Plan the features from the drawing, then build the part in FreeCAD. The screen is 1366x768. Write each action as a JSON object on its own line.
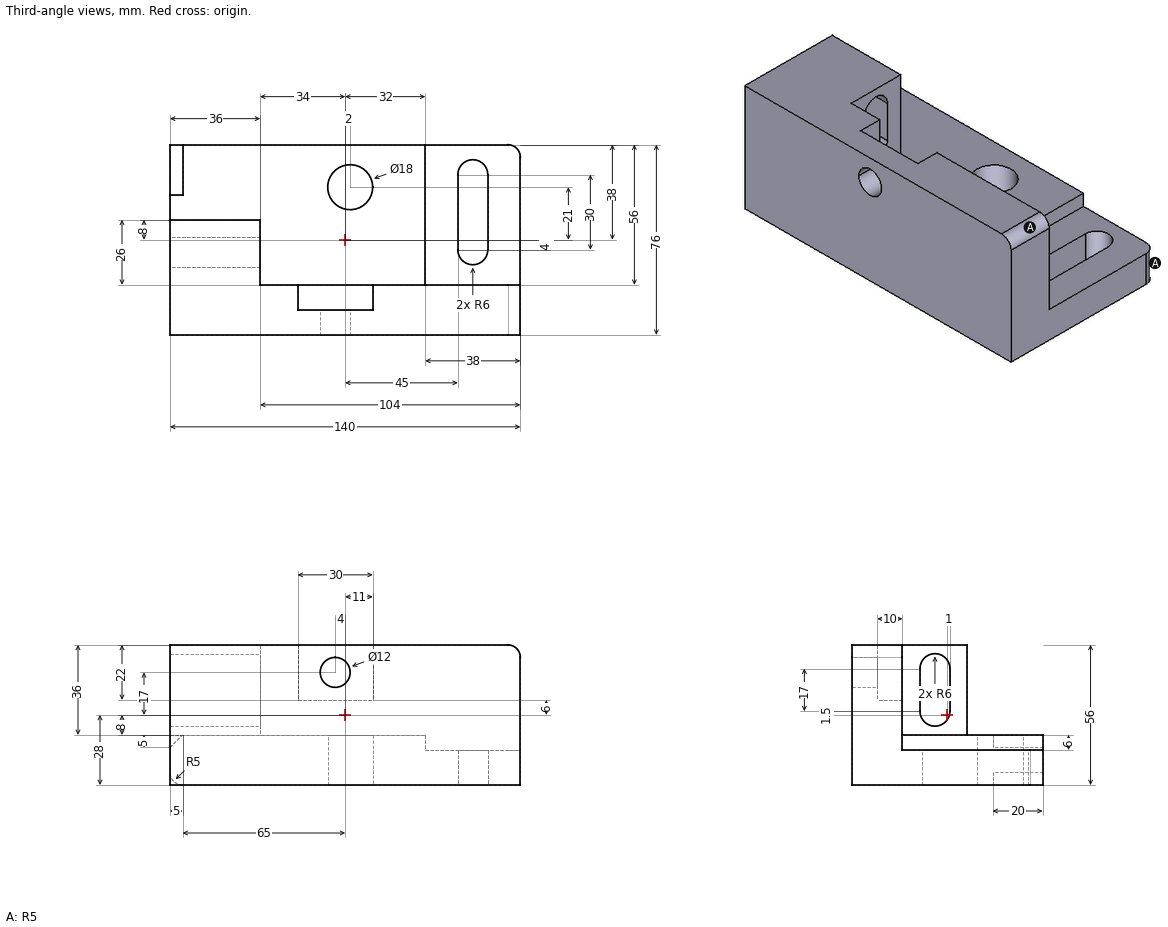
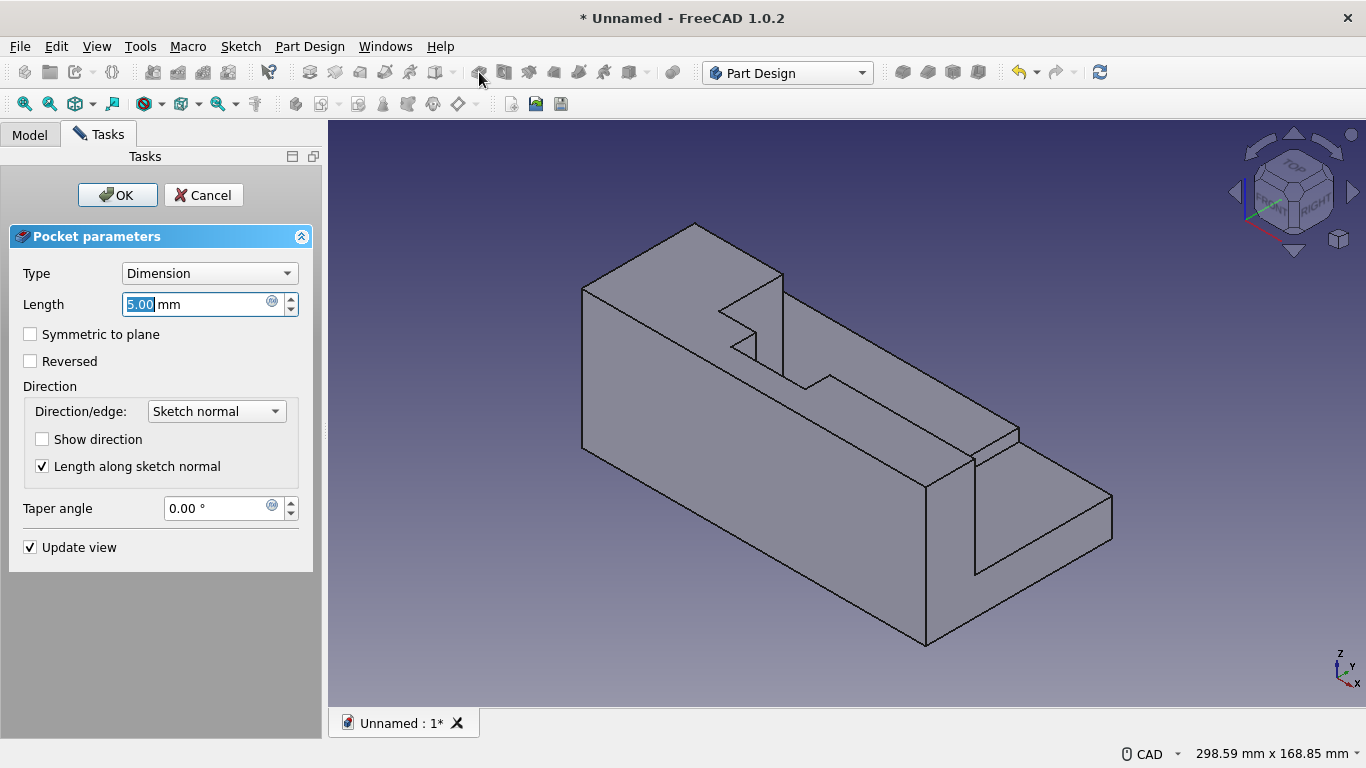
{"action": "type", "text": "6"}
{"action": "key", "text": "Tab"}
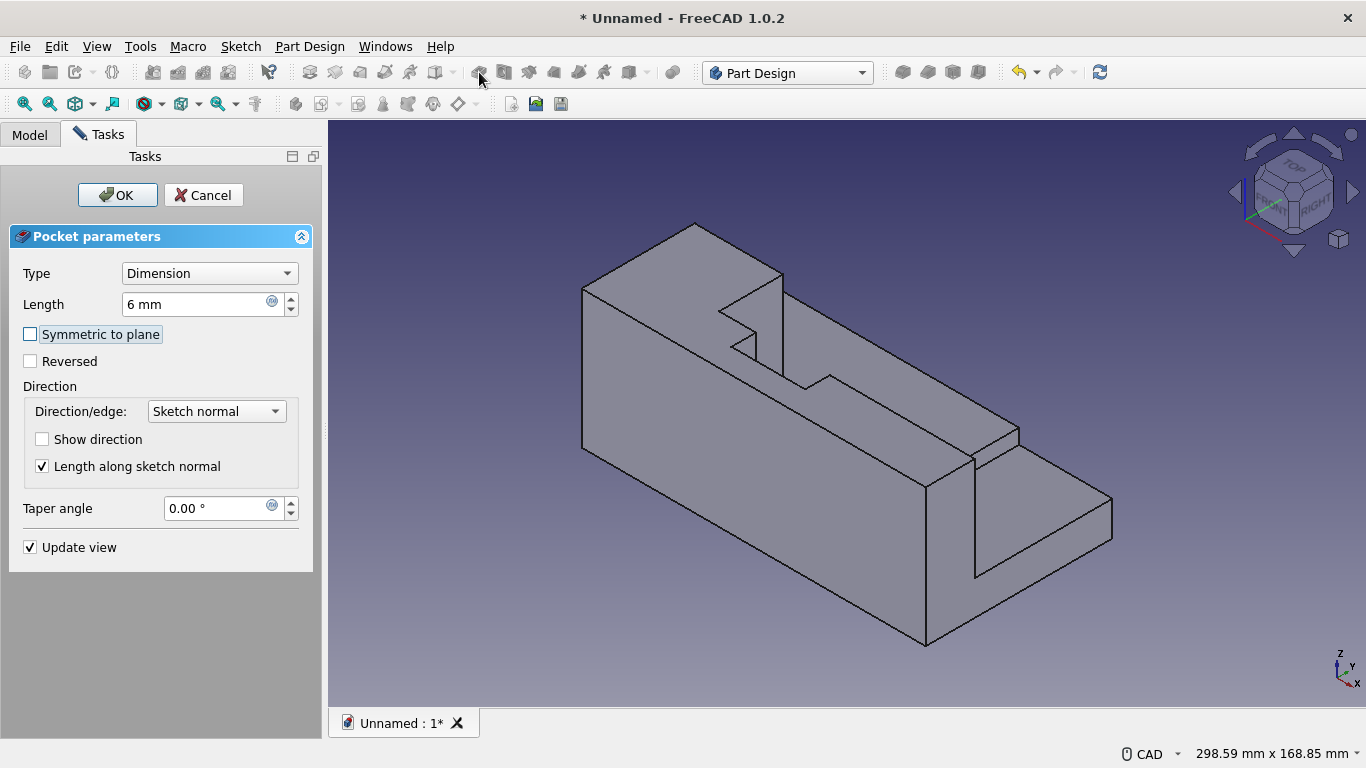
{"action": "left_click", "coordinate": [118, 195]}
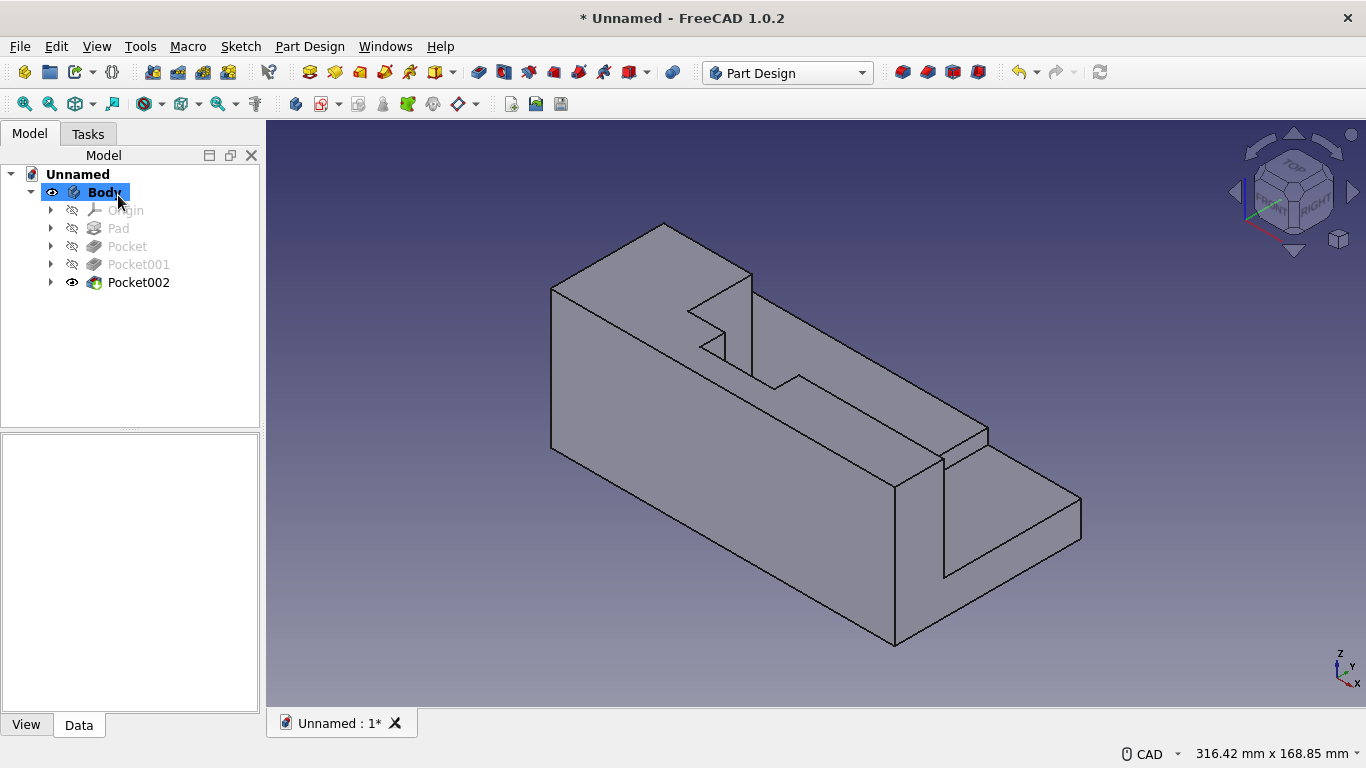
{"action": "key", "text": "2"}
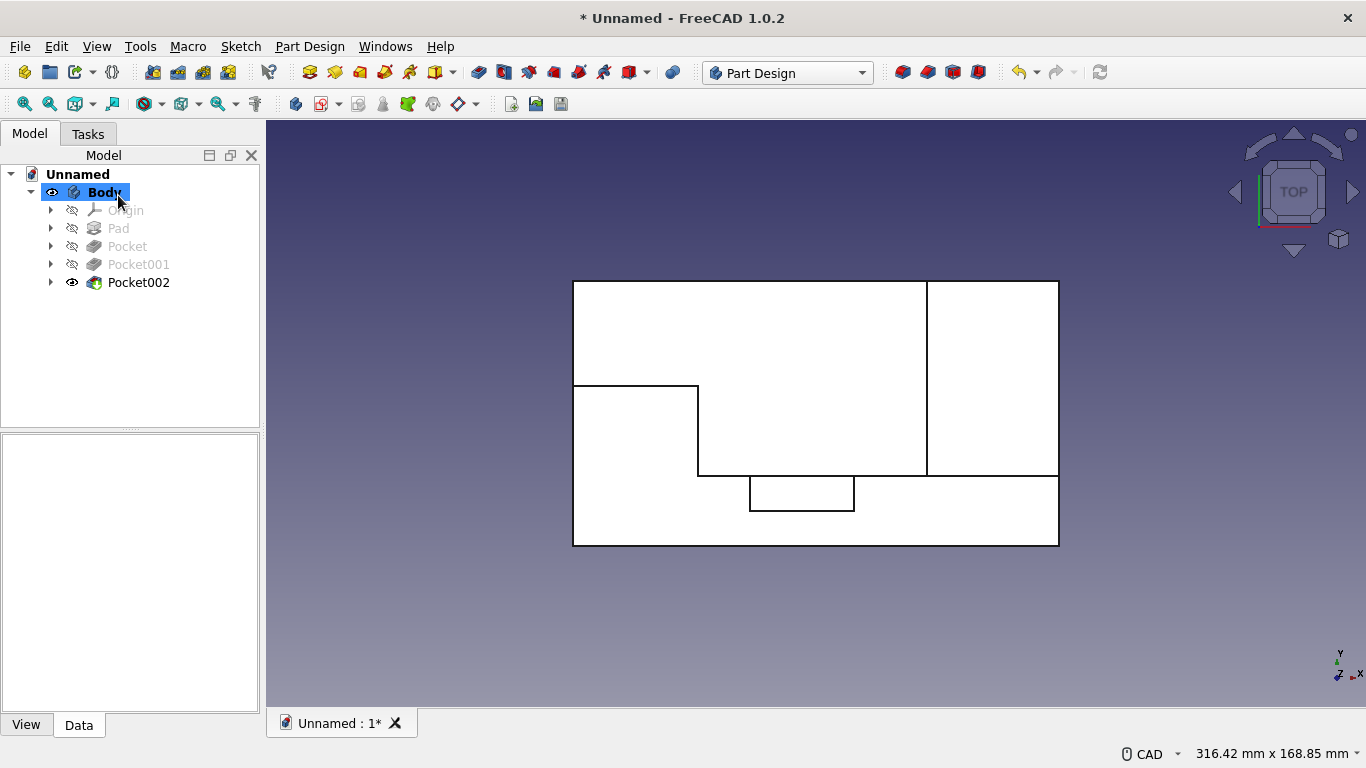
{"action": "left_click", "coordinate": [801, 378]}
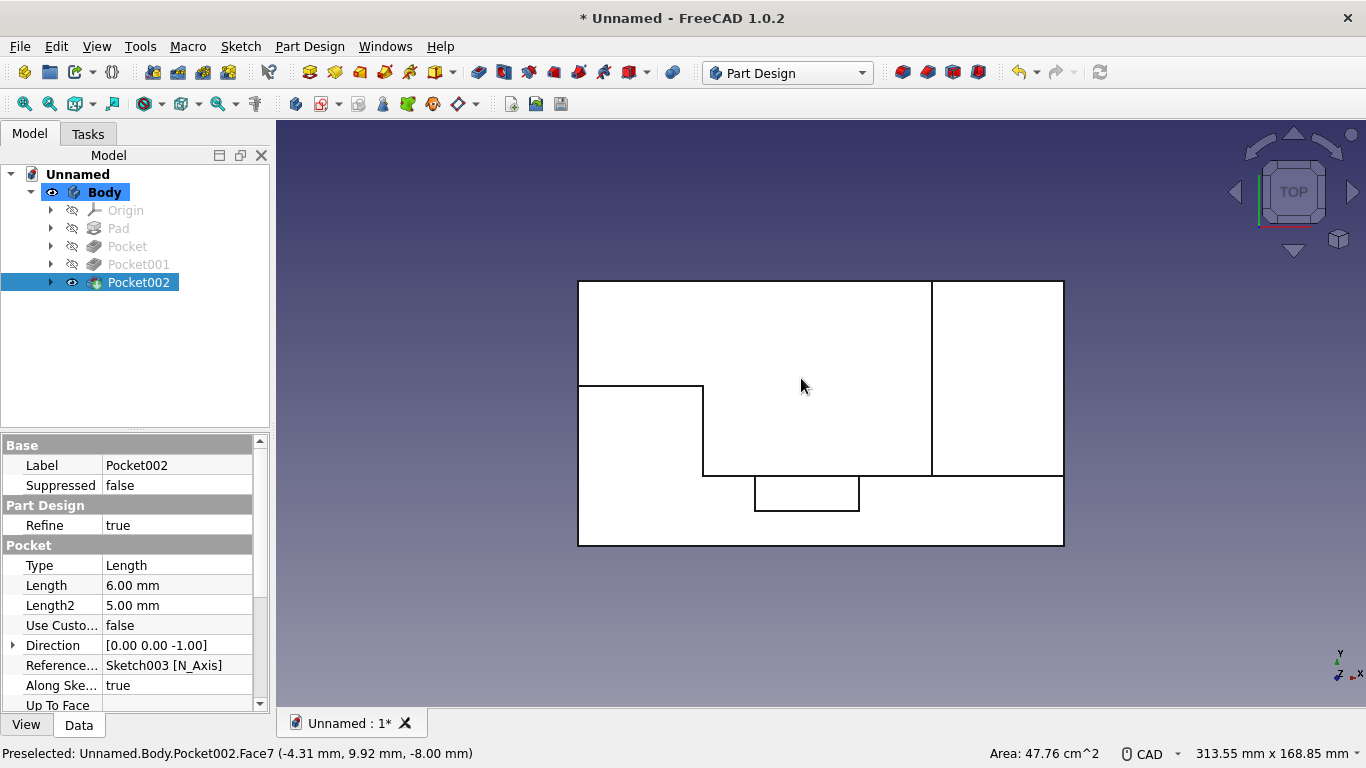
{"action": "left_click", "coordinate": [320, 104]}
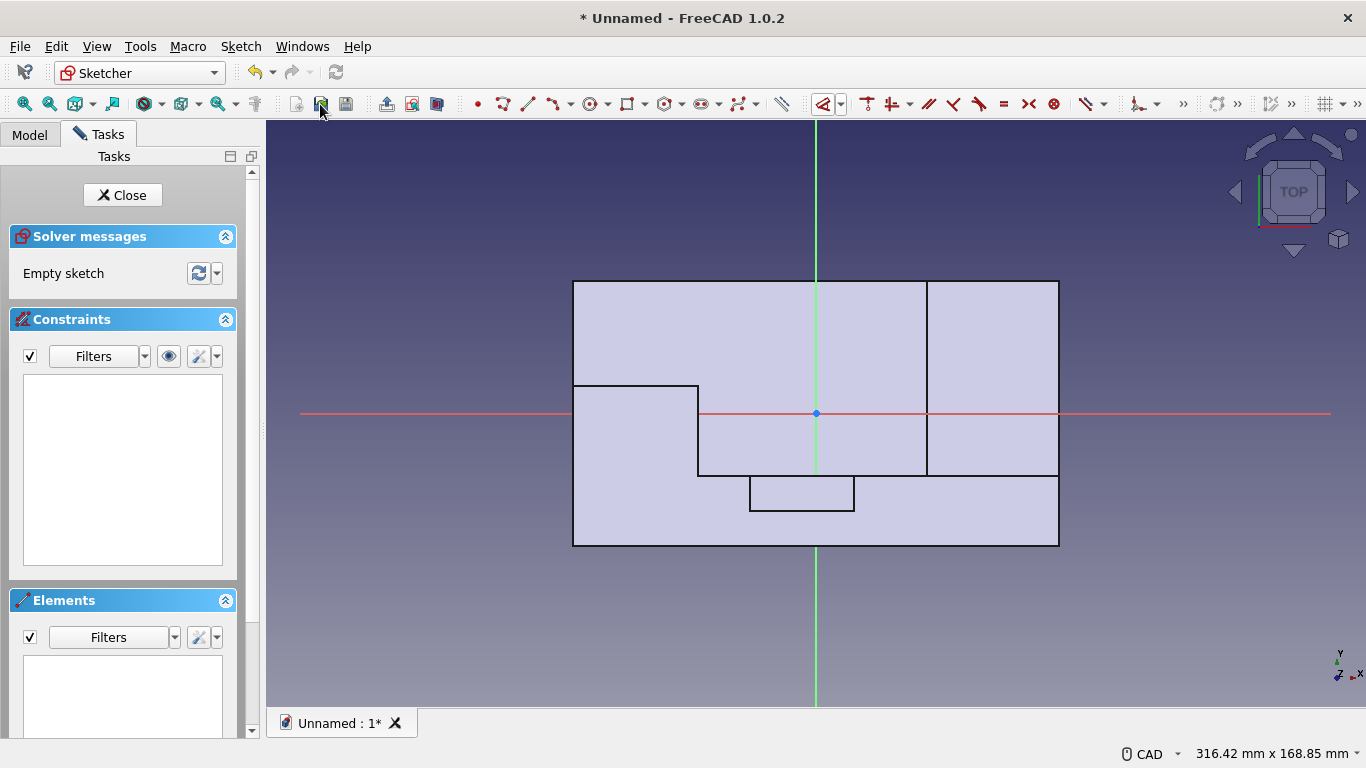
{"action": "scroll", "coordinate": [993, 353], "scroll_direction": "up", "scroll_amount": 5}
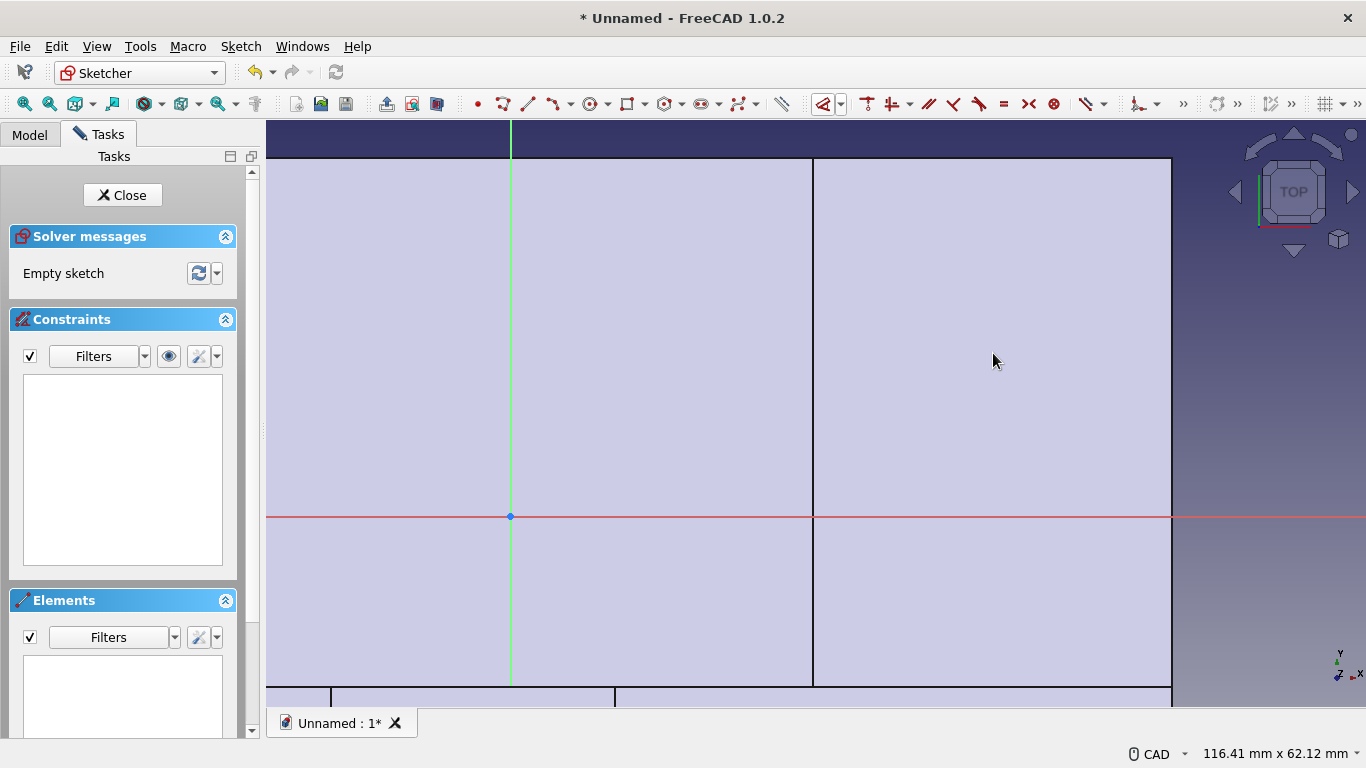
{"action": "left_click", "coordinate": [700, 104]}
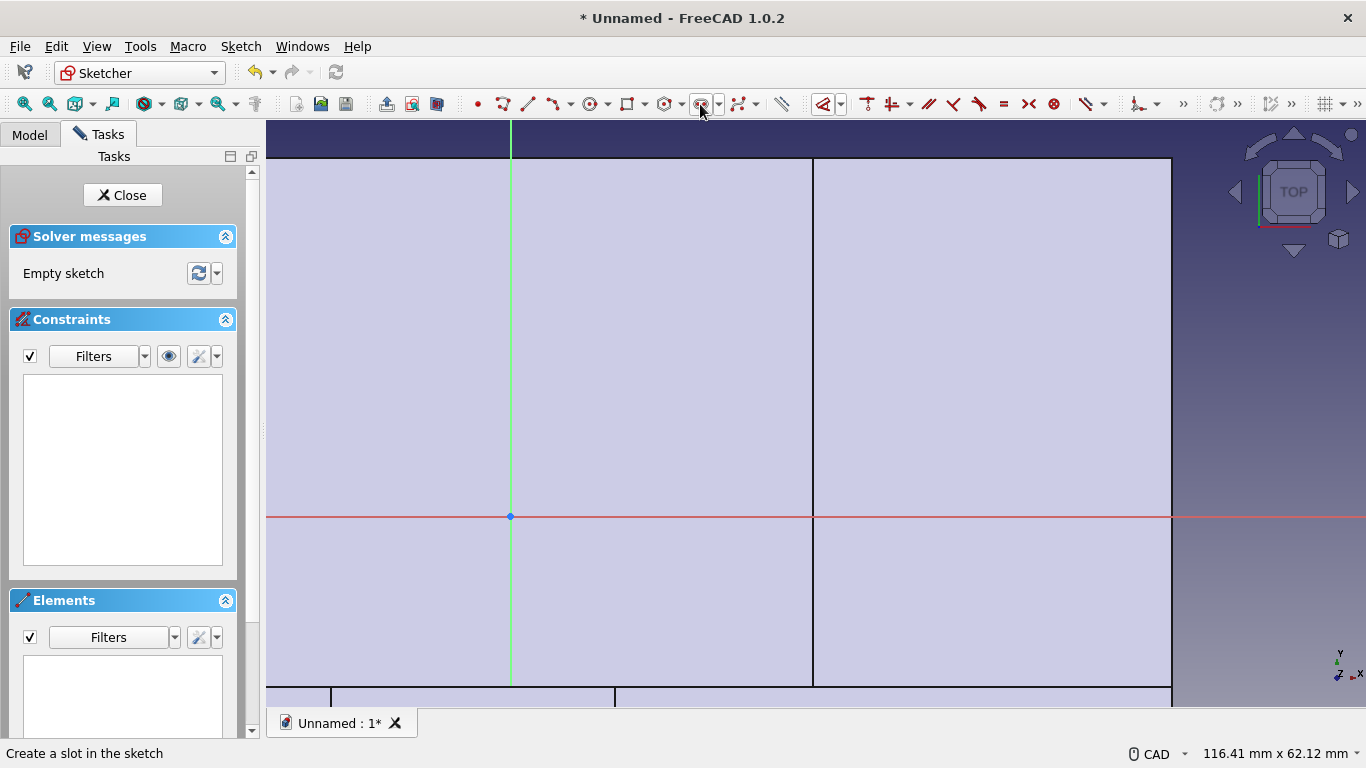
{"action": "left_click", "coordinate": [993, 555]}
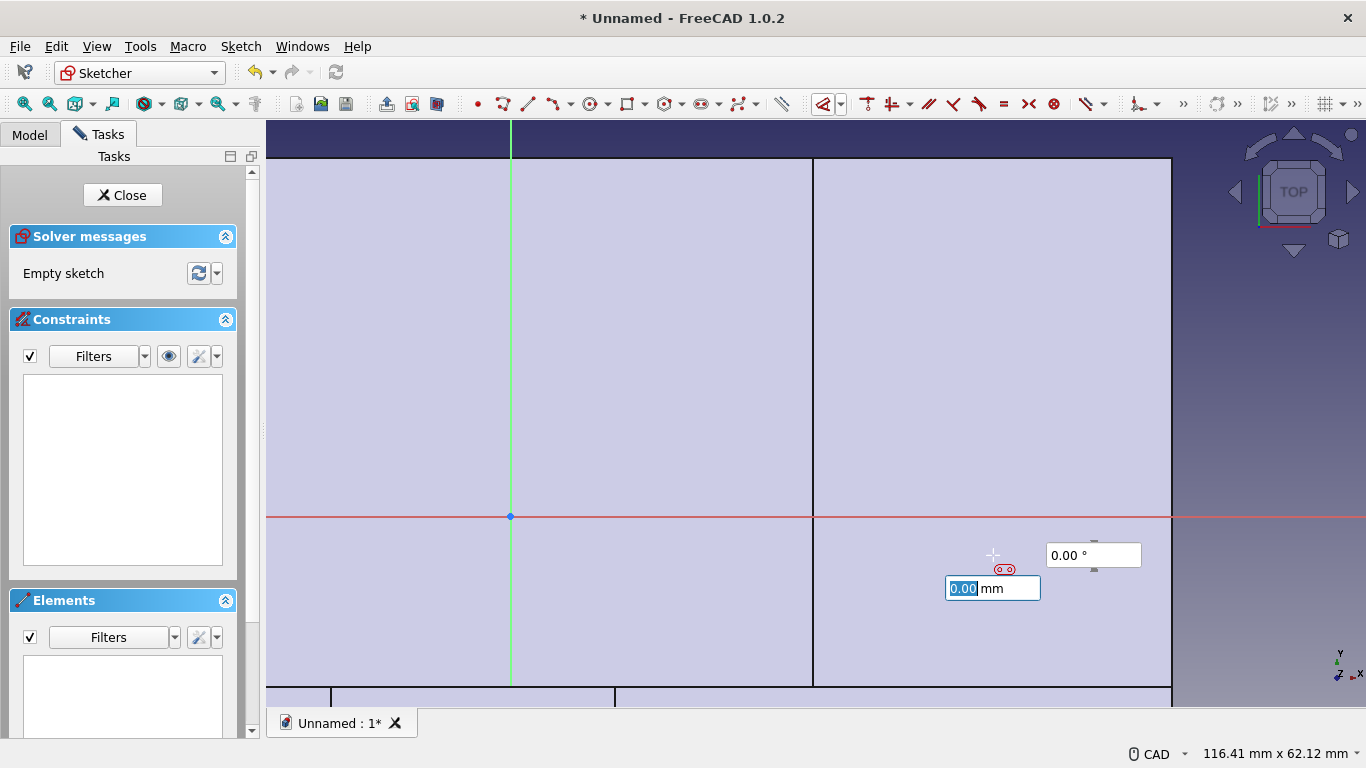
{"action": "left_click", "coordinate": [993, 271]}